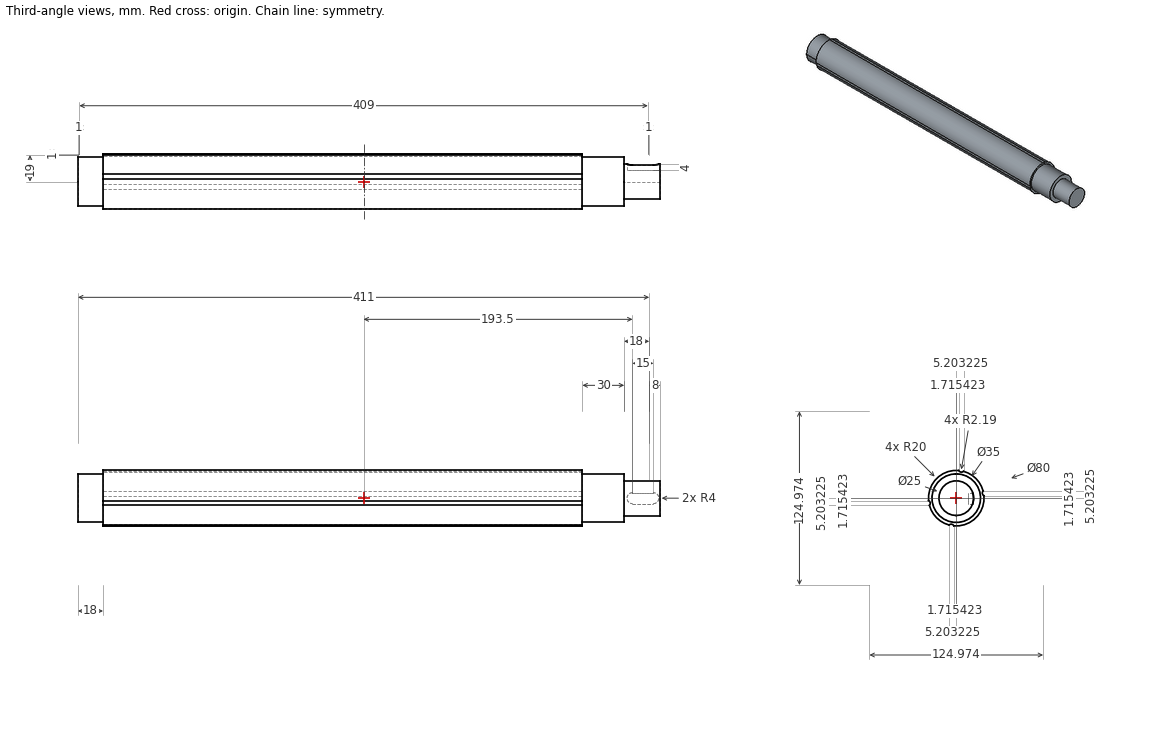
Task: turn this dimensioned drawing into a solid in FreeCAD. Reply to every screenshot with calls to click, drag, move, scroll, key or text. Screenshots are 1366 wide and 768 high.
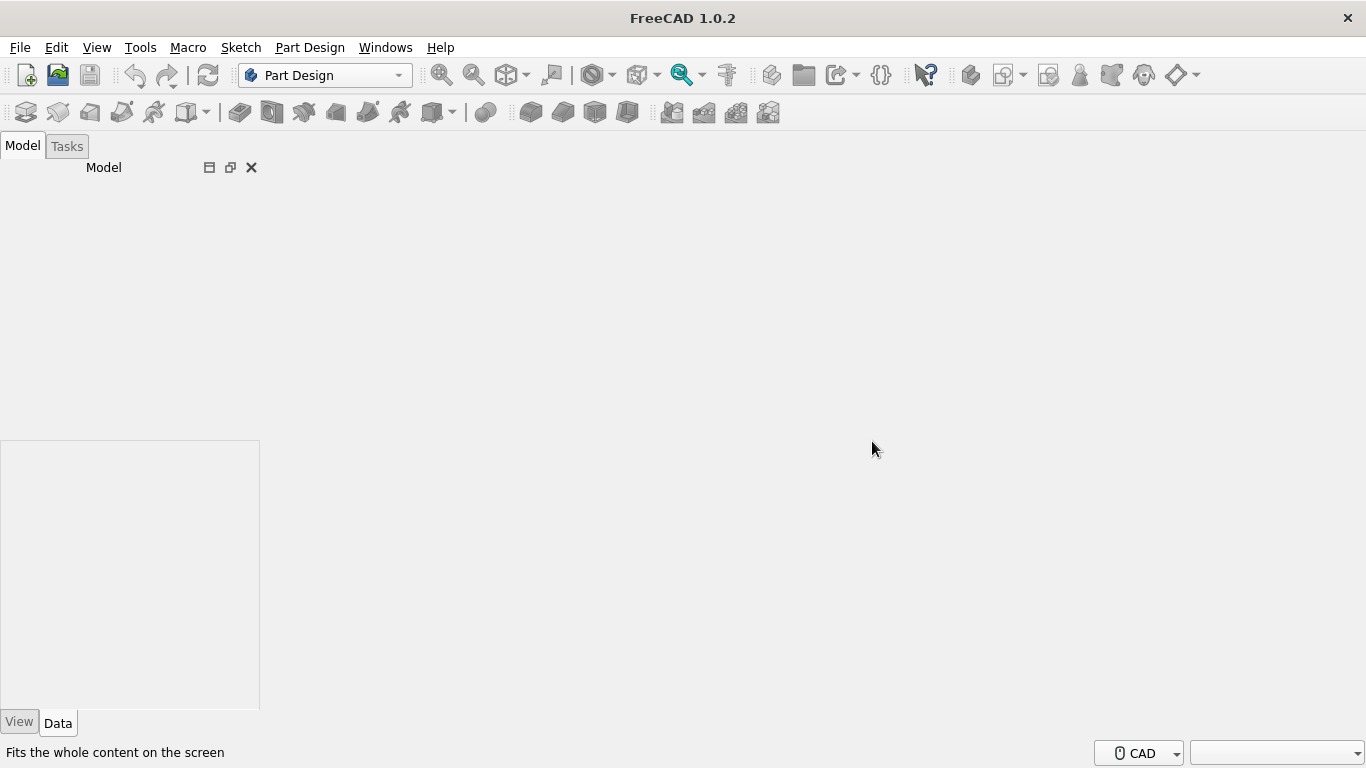
key(ctrl+n)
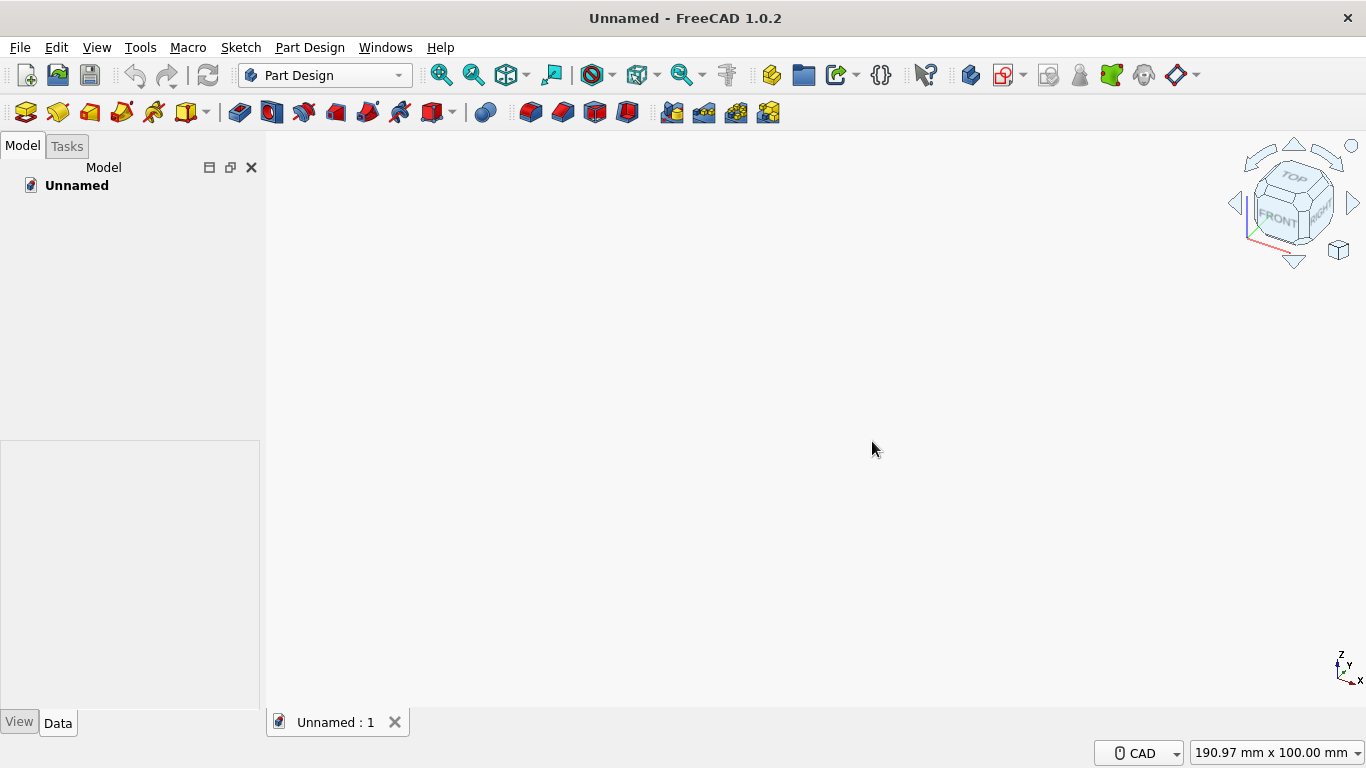
click(1004, 76)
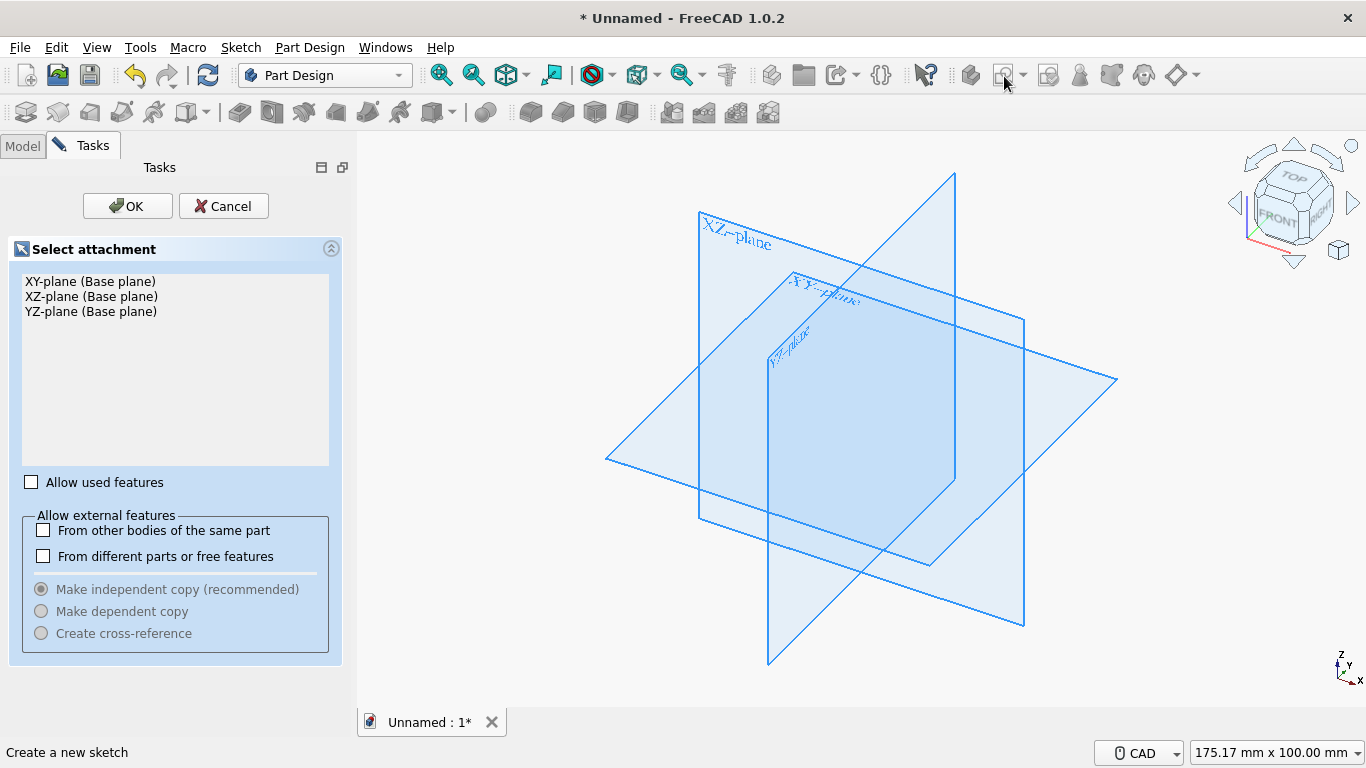
click(82, 282)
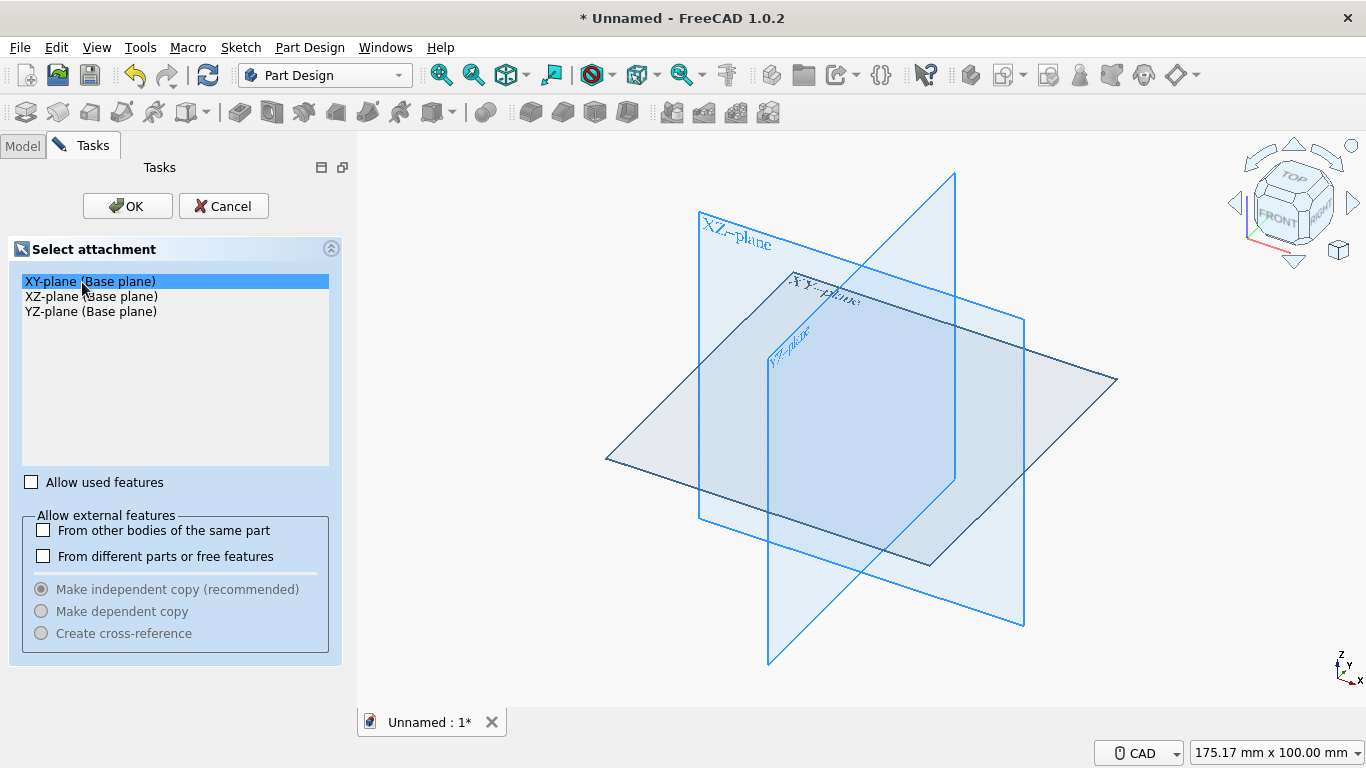
click(128, 206)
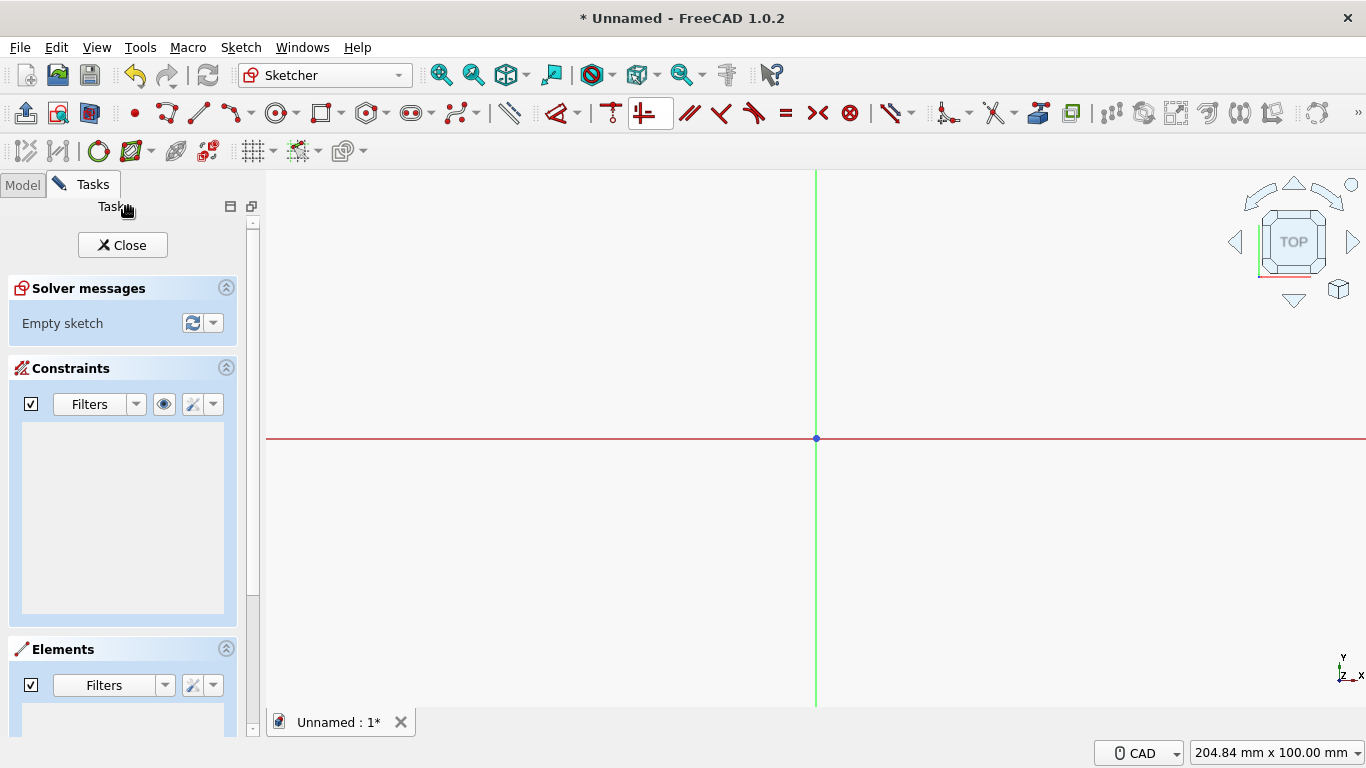
scroll(718, 462, down, 6)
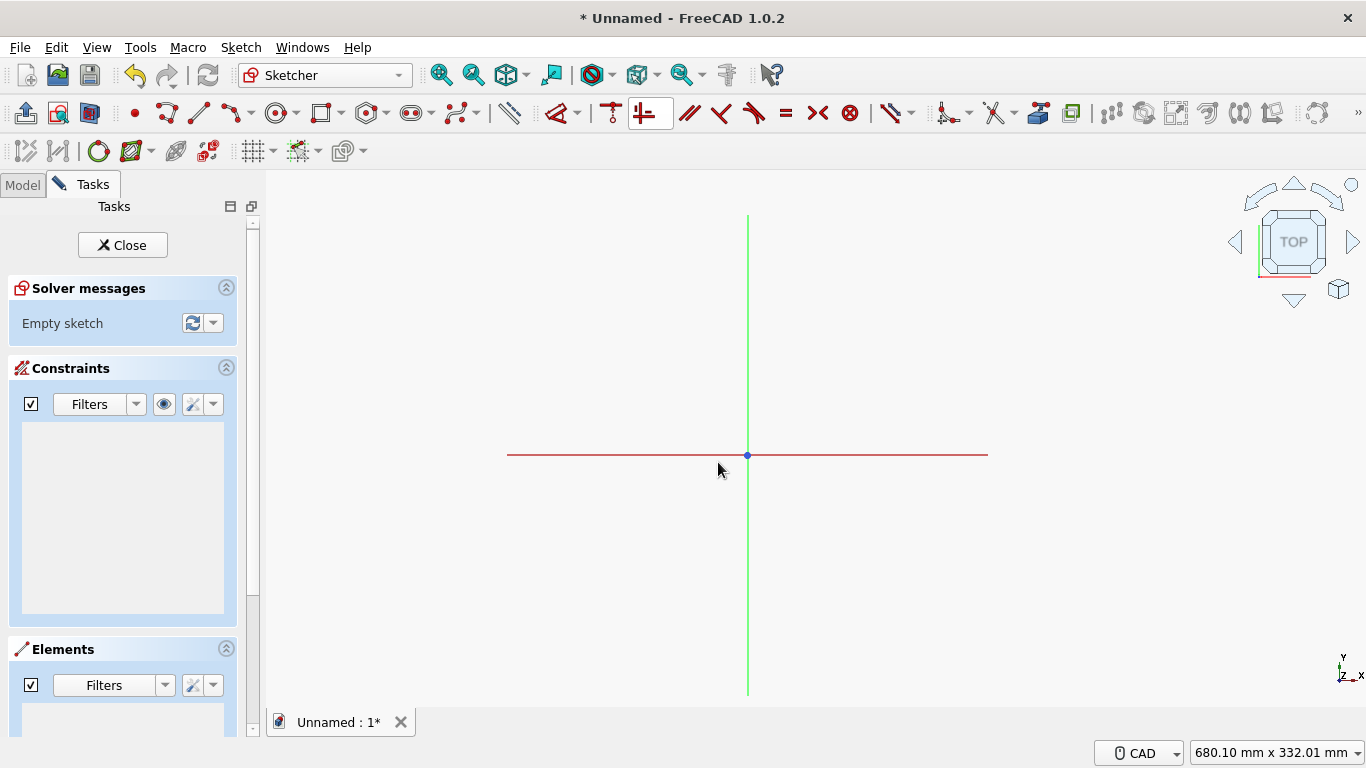
key(g)
key(m)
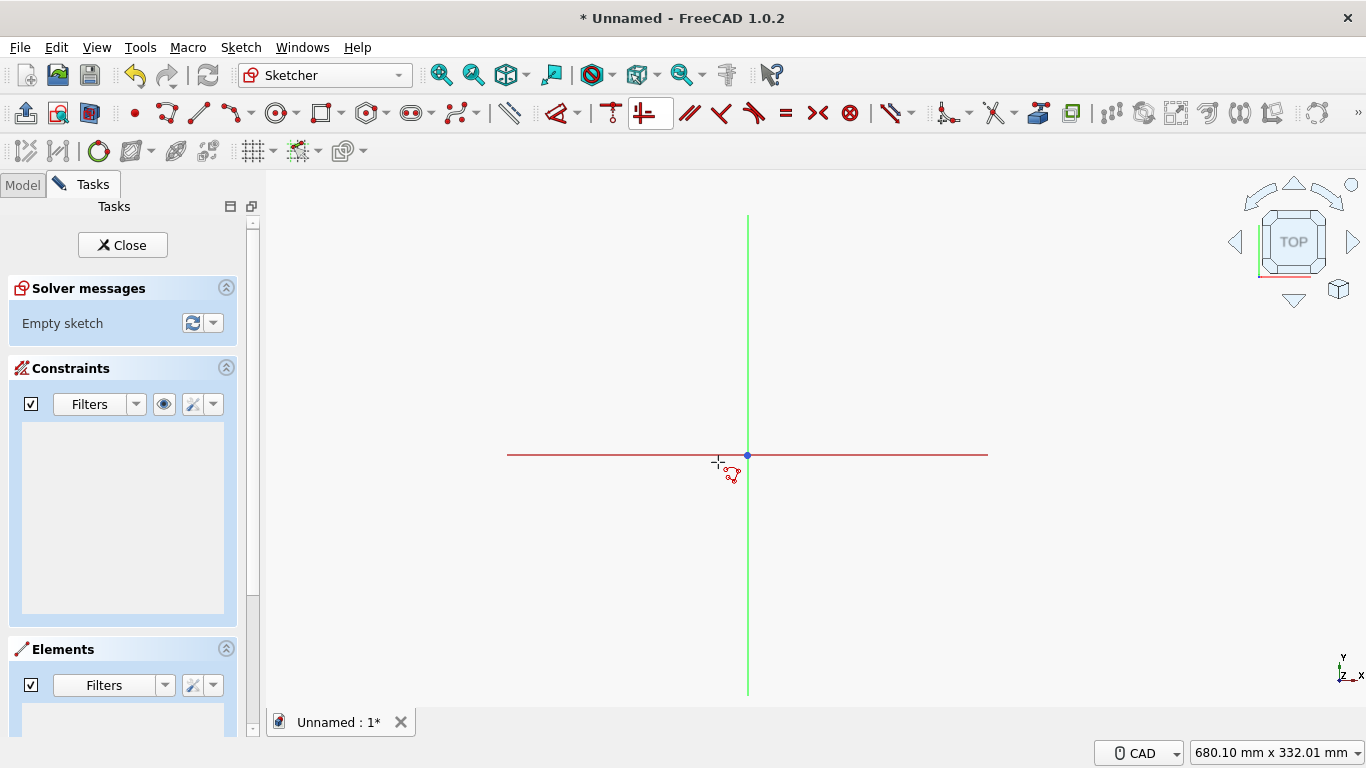
click(1079, 423)
click(417, 423)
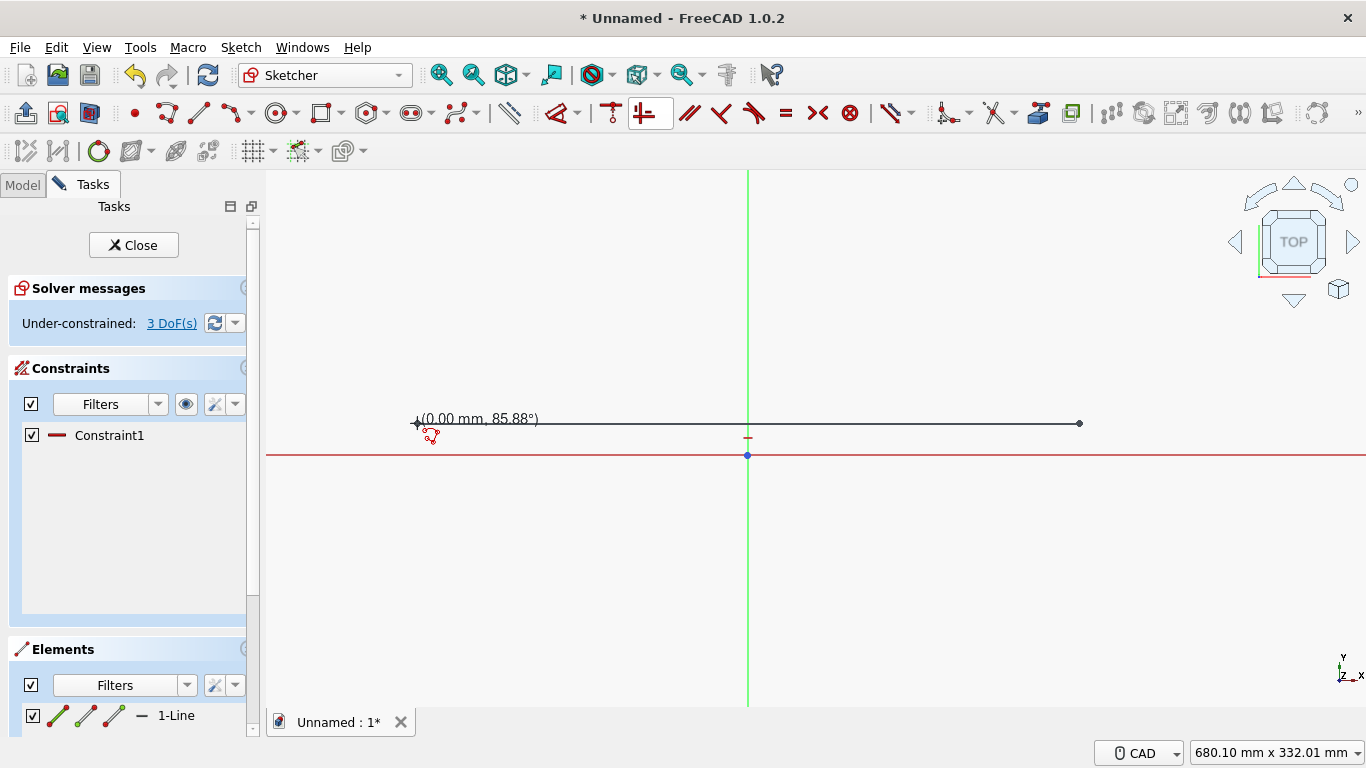
scroll(415, 425, up, 10)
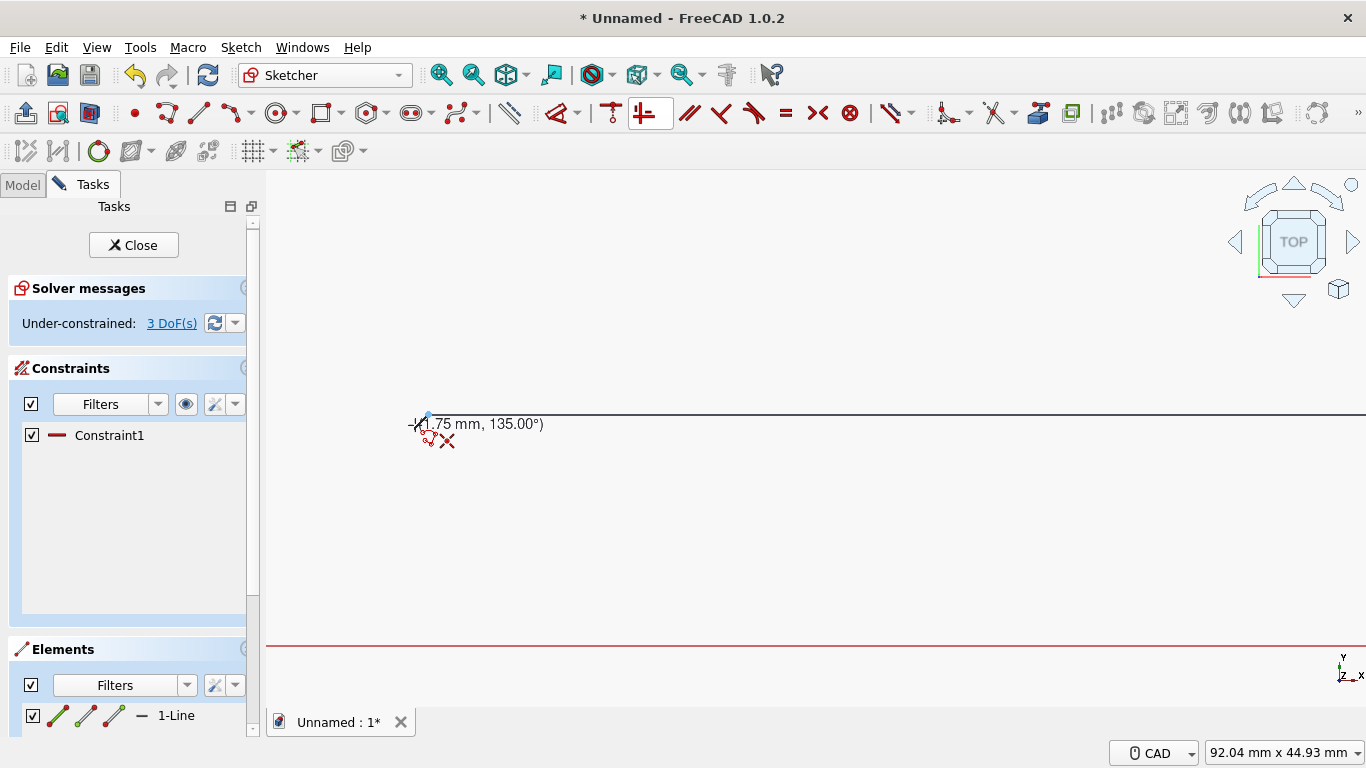
click(417, 419)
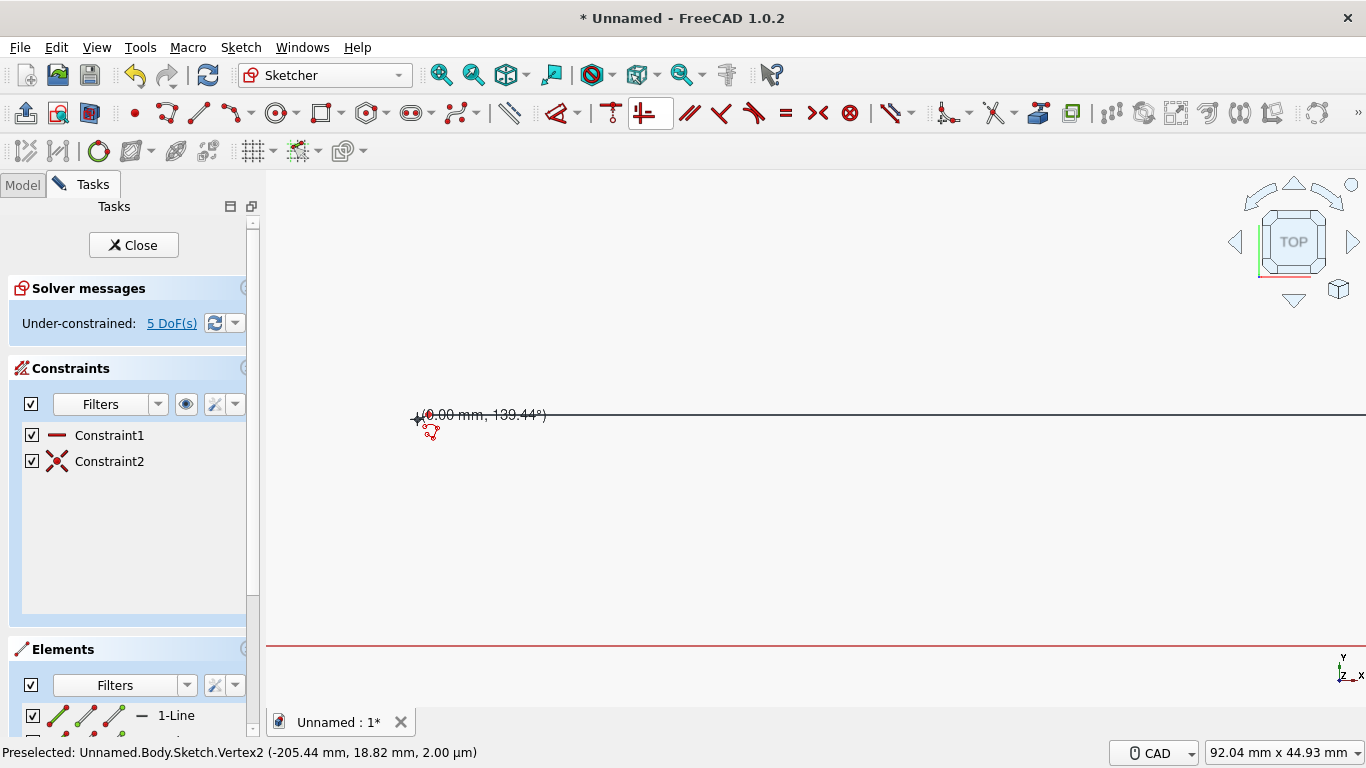
scroll(415, 425, down, 10)